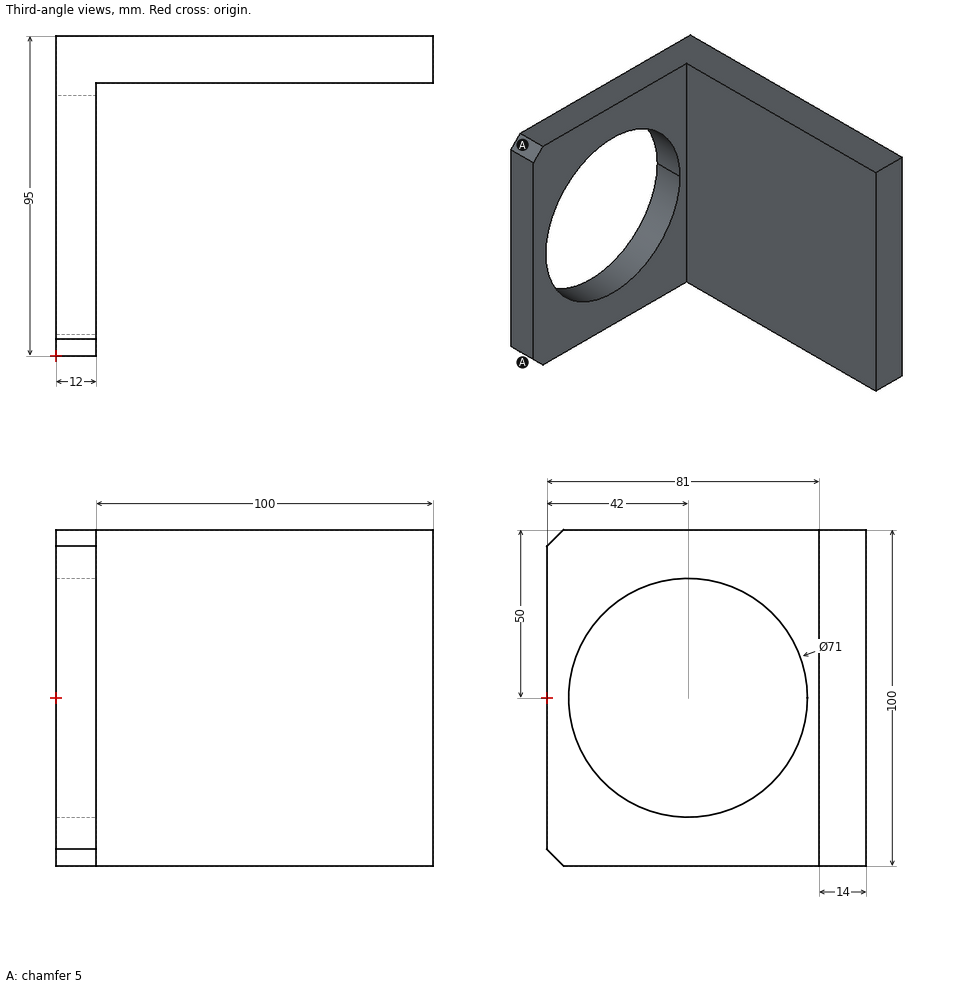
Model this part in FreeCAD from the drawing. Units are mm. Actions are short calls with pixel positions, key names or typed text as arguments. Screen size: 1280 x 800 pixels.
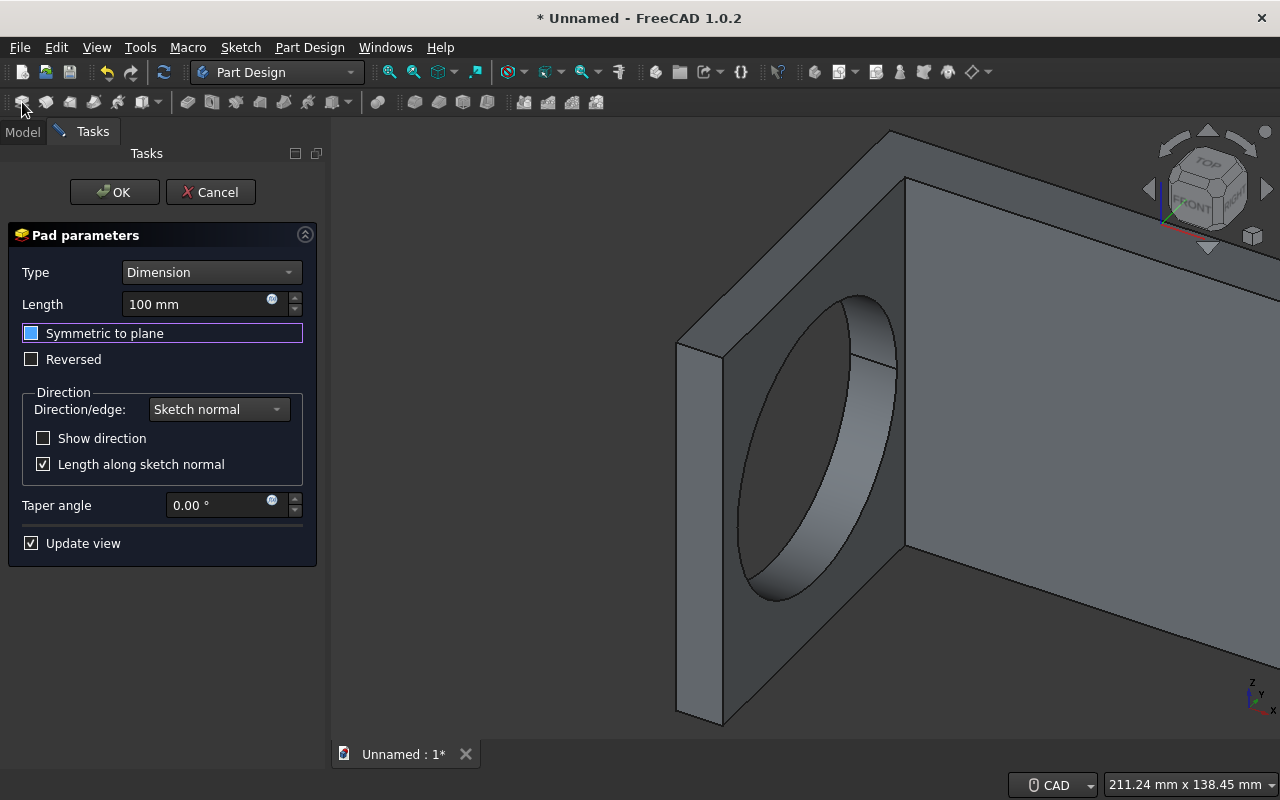
click(115, 192)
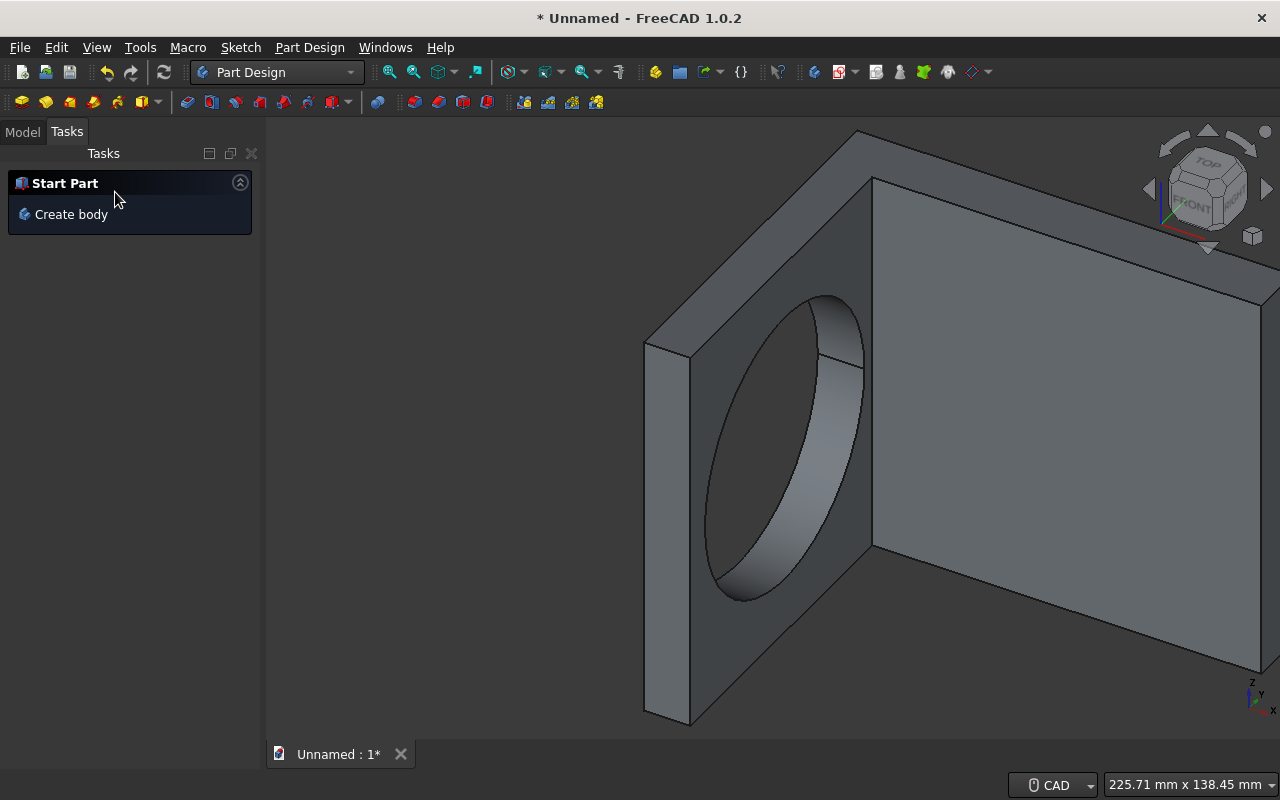
click(390, 72)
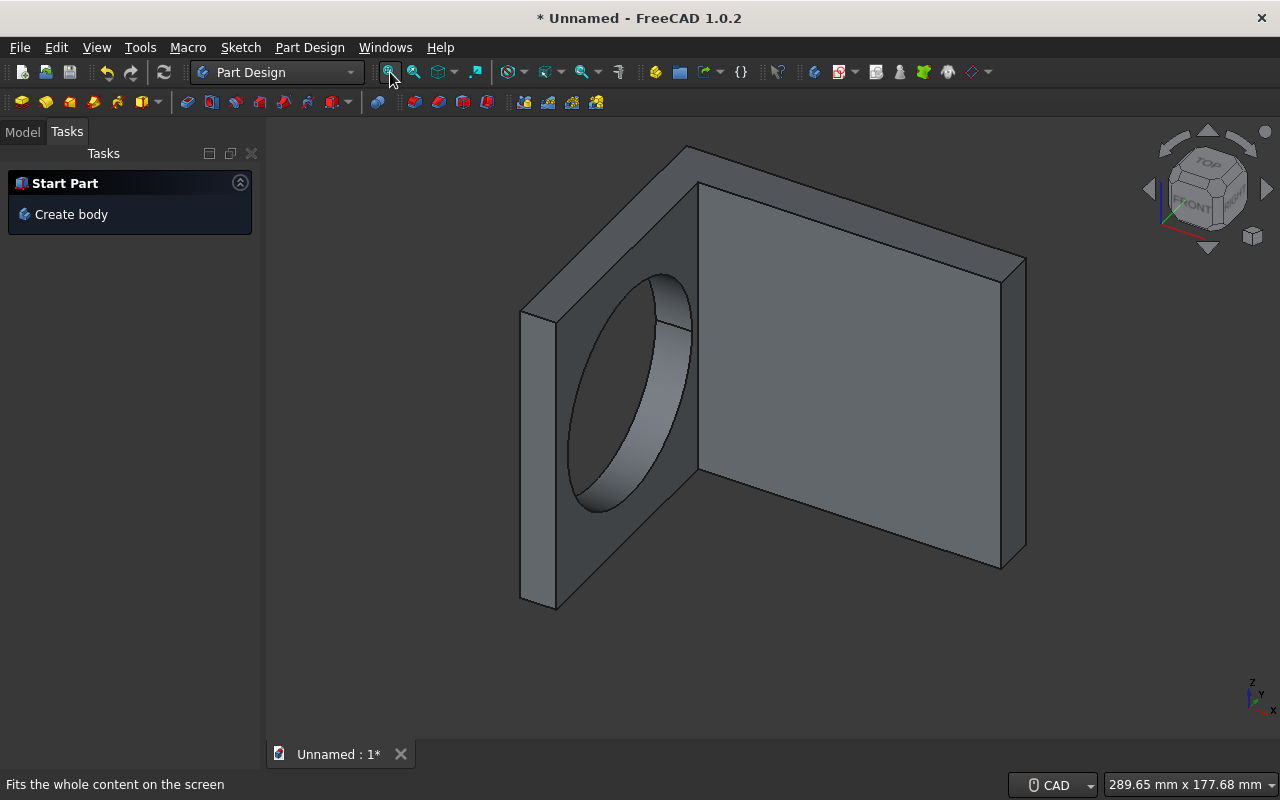
click(538, 316)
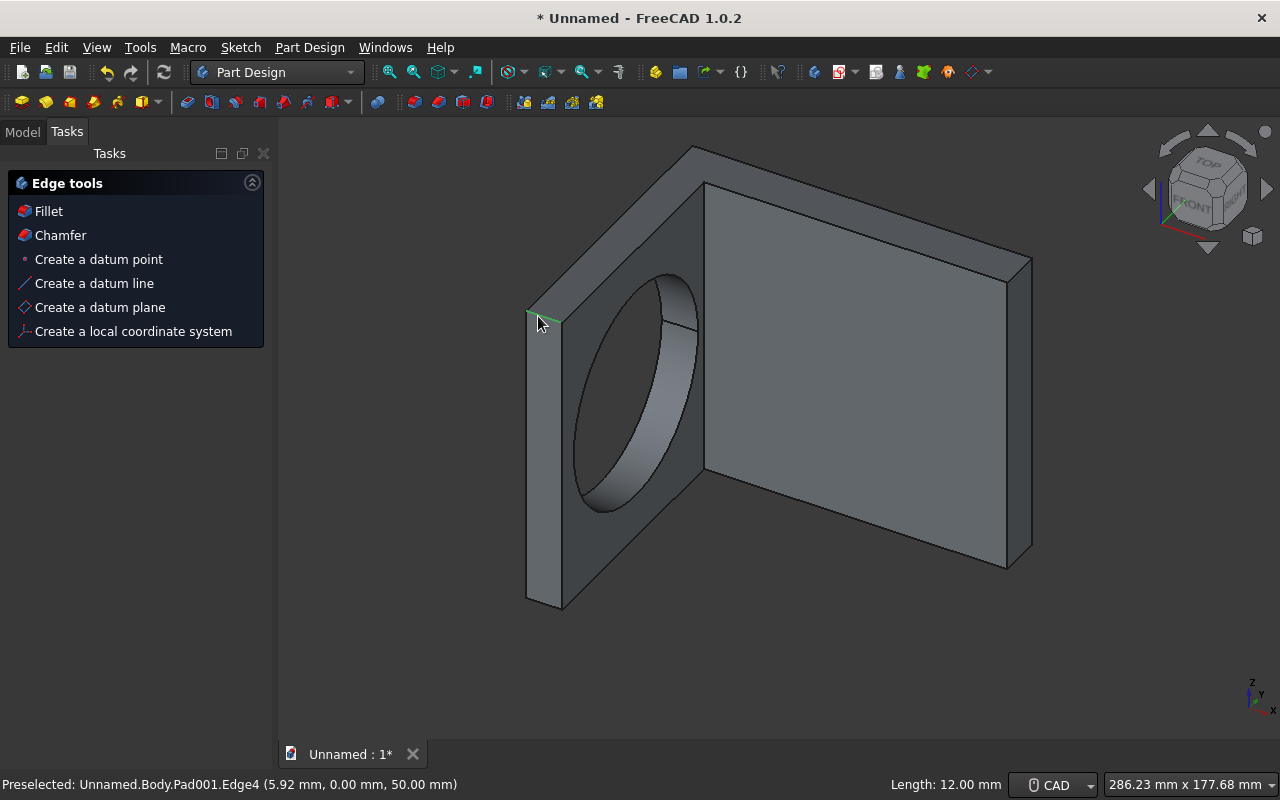
key(0)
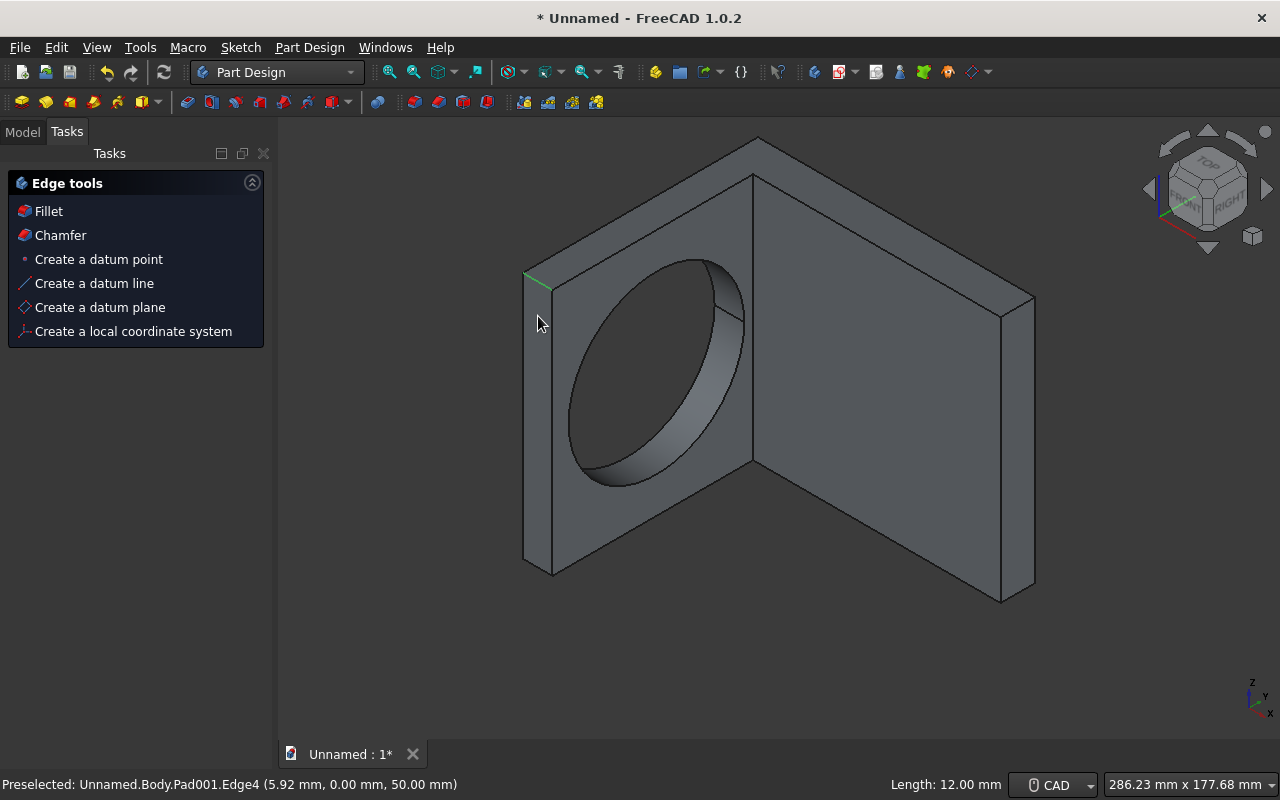
key(2)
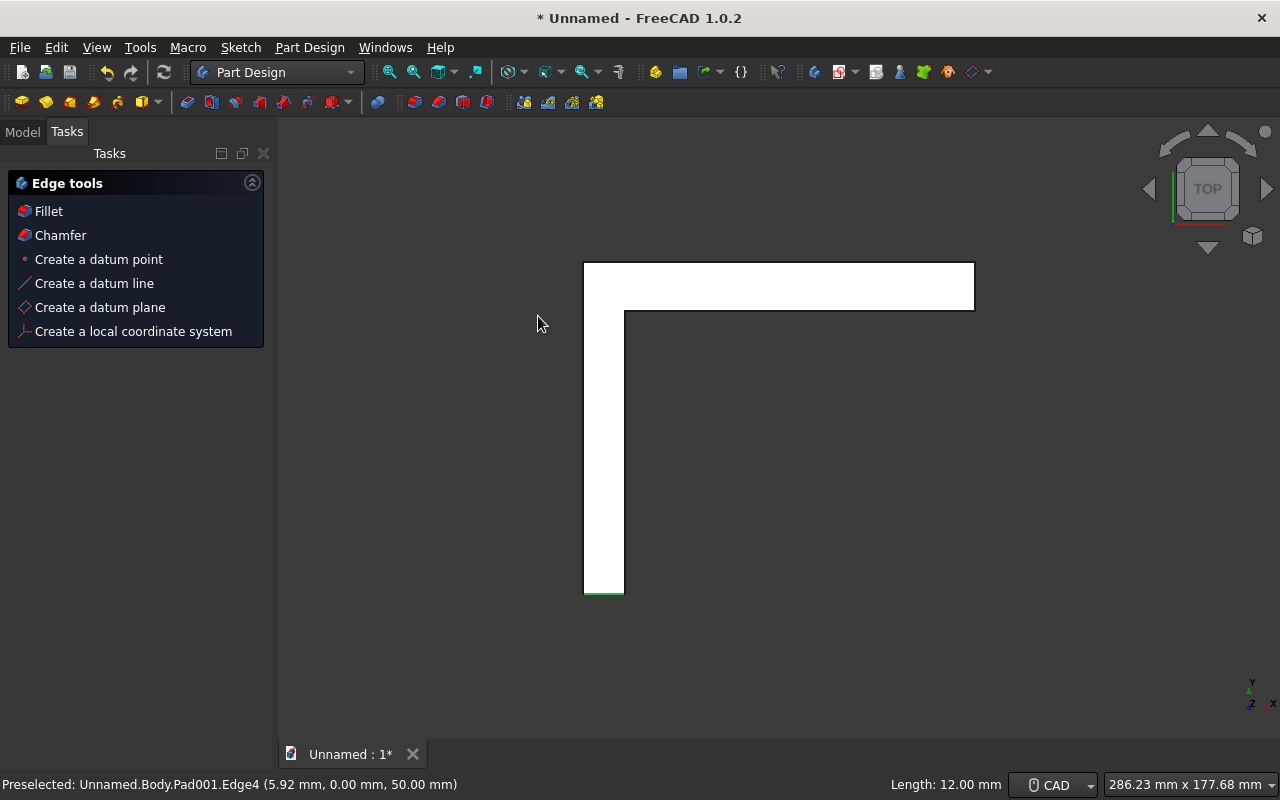
key(1)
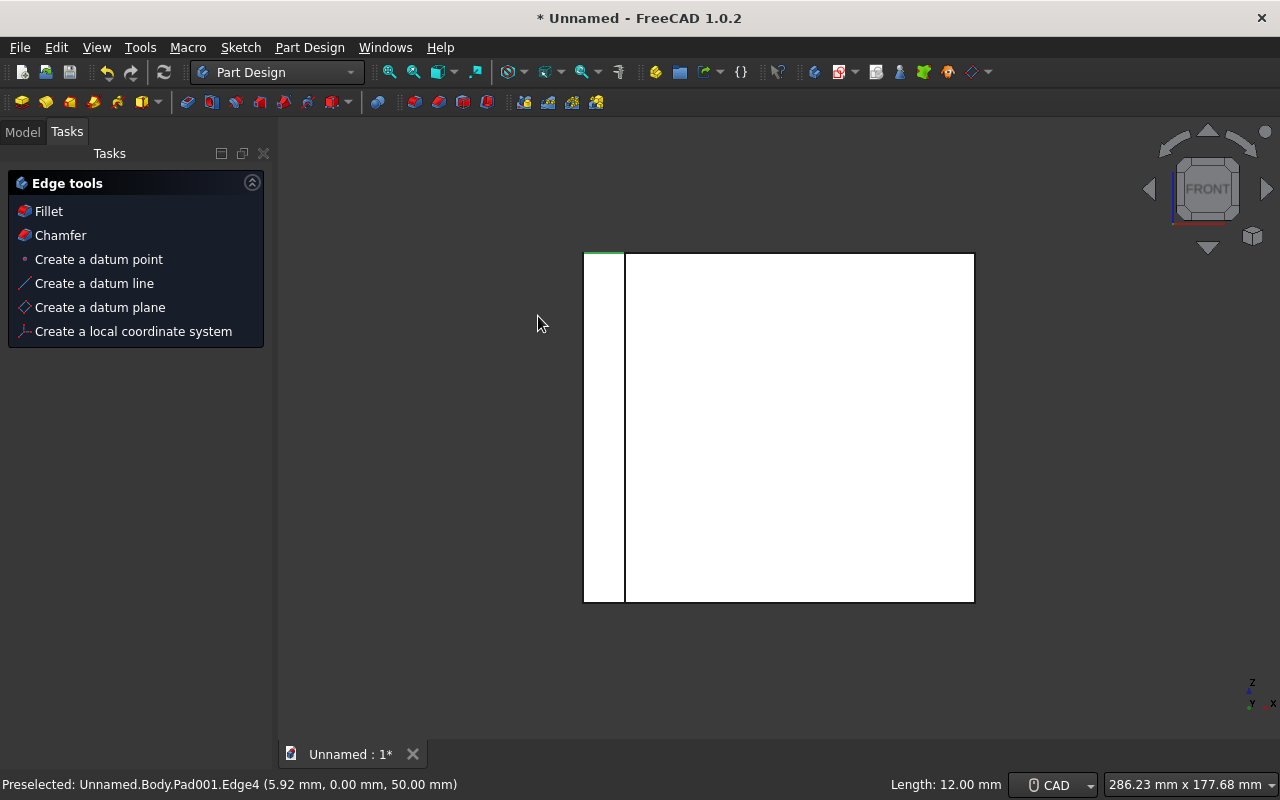
click(604, 602, ctrl)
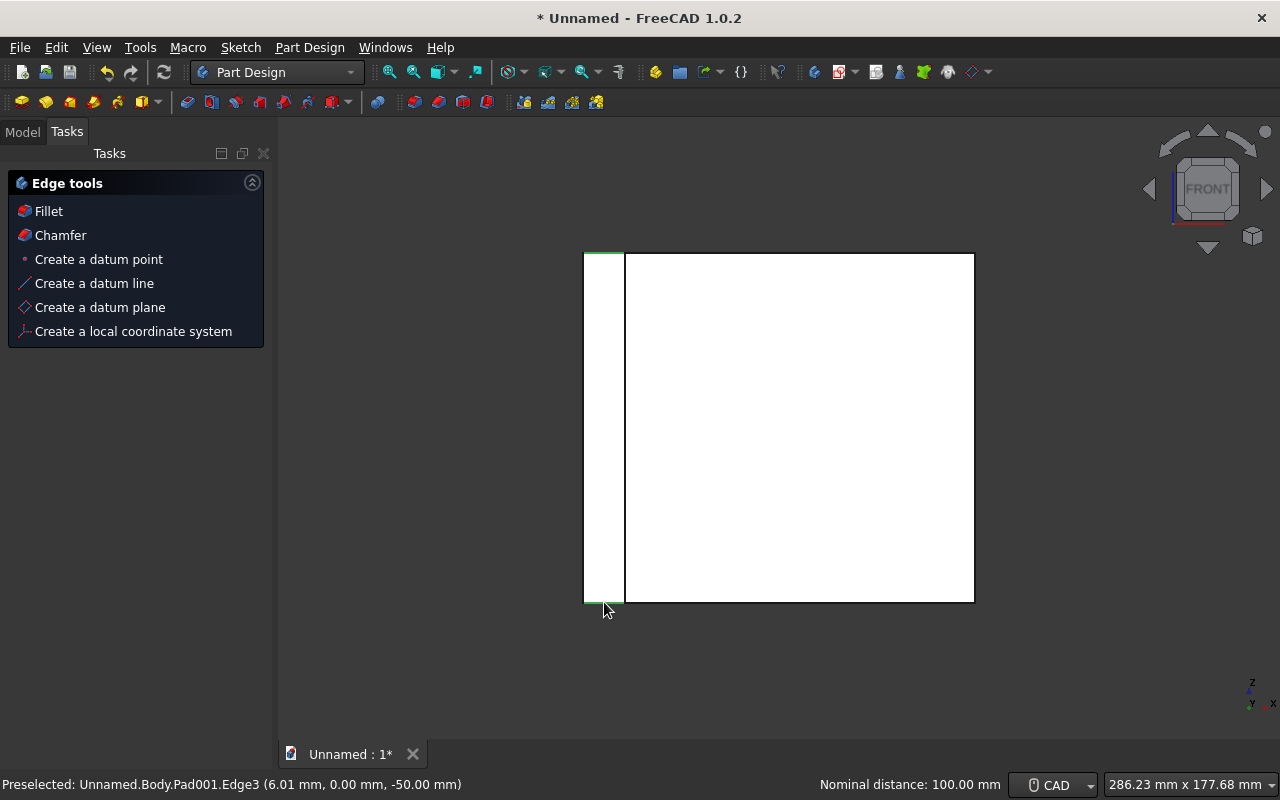
click(440, 102)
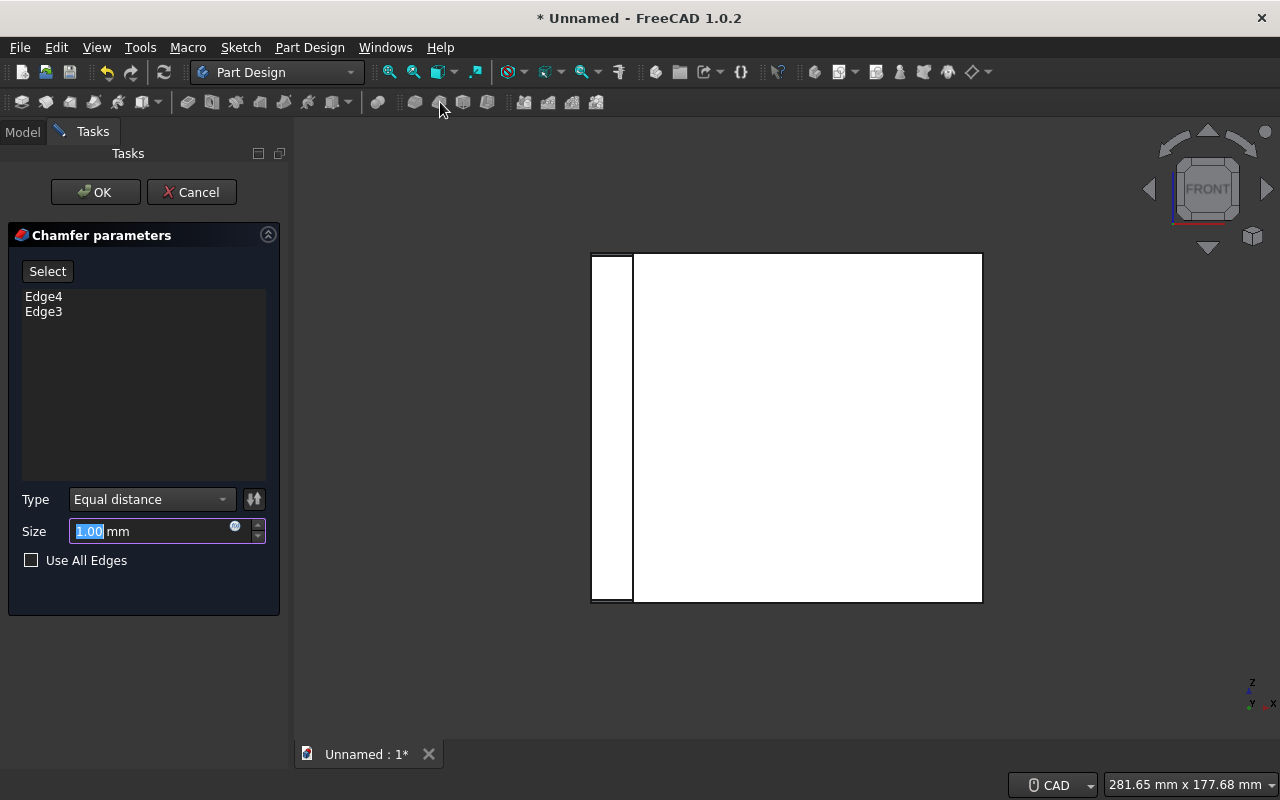
text(5)
key(Tab)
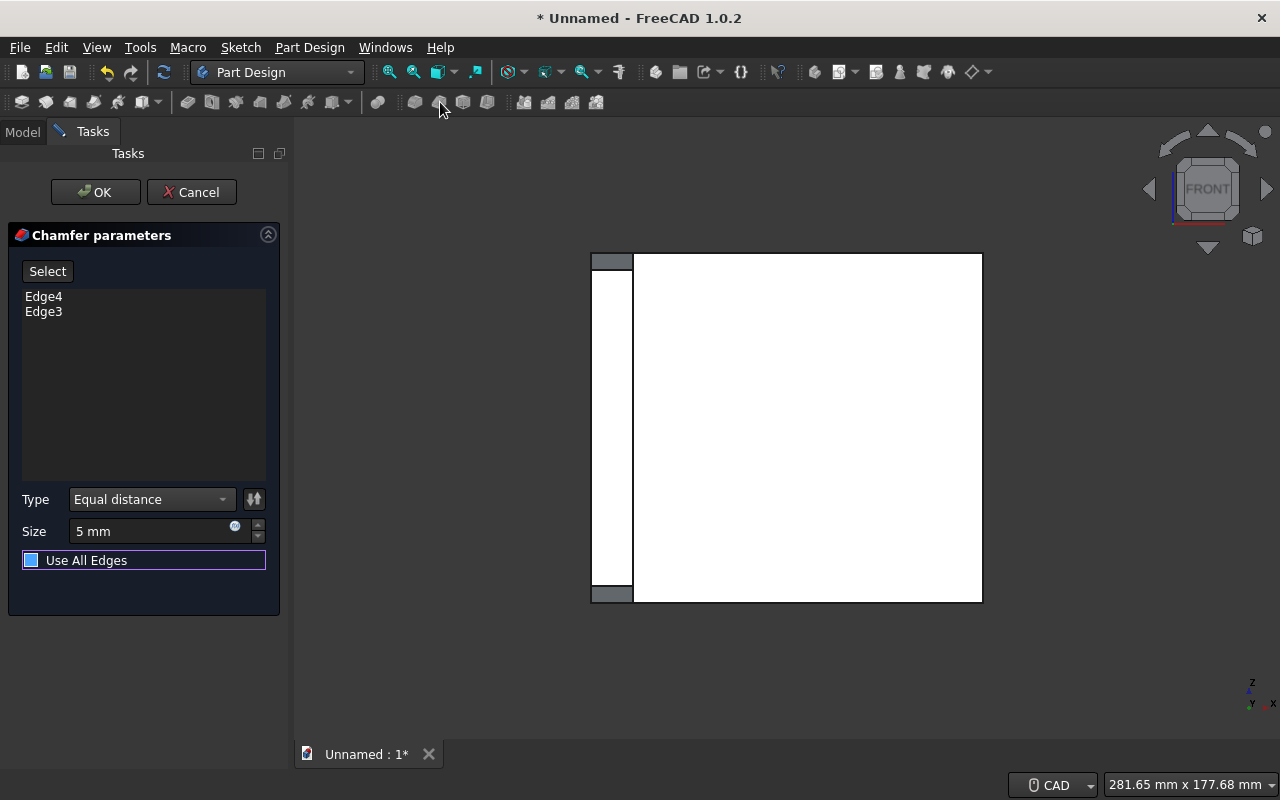
click(96, 192)